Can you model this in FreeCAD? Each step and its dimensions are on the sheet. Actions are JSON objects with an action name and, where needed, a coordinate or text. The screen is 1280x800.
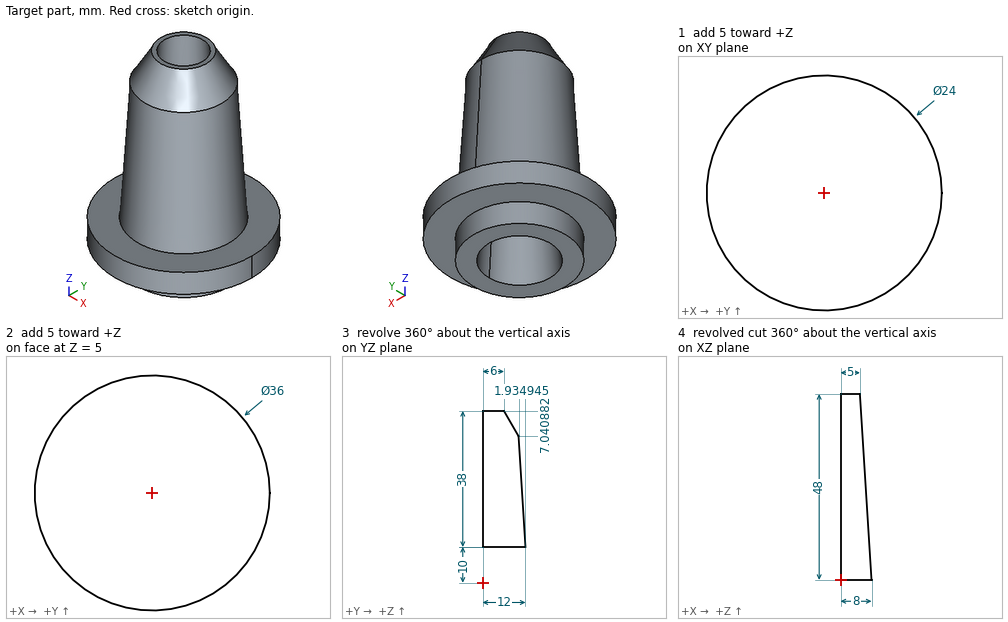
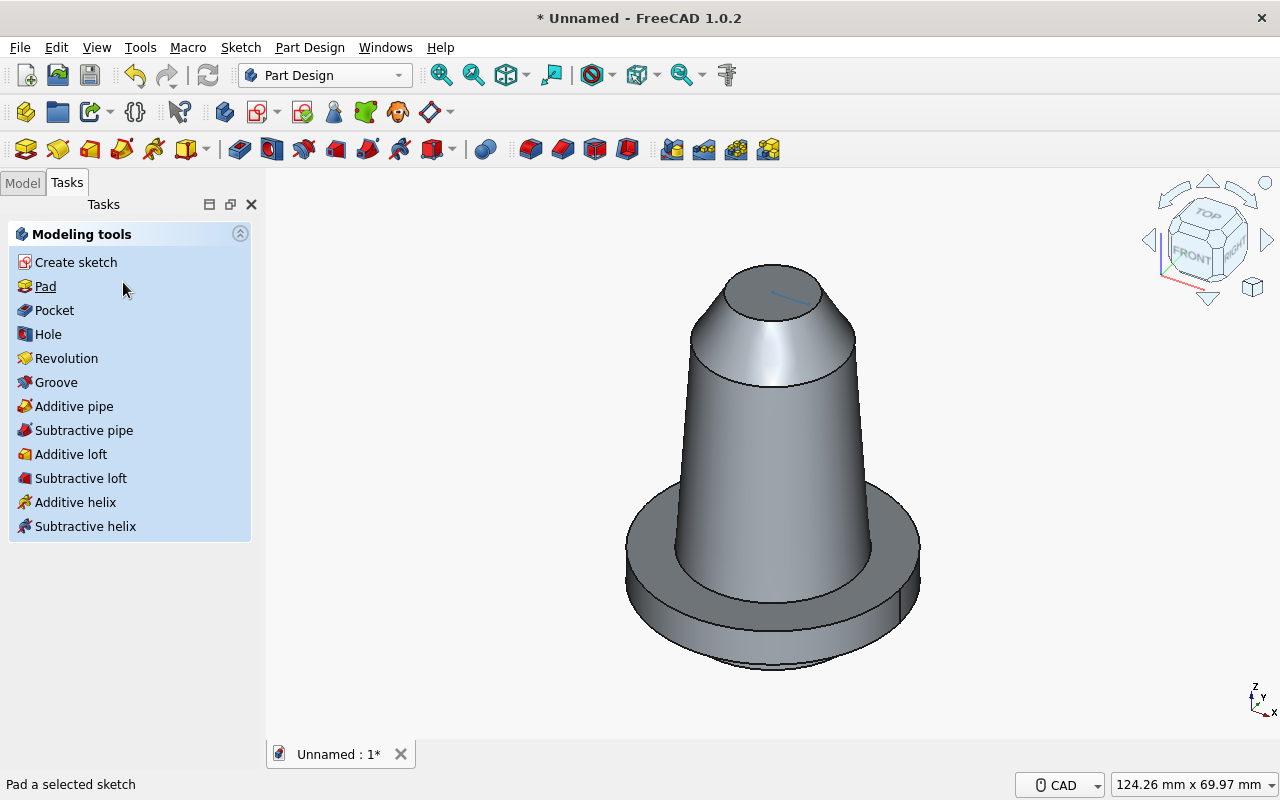
{"action": "left_click", "coordinate": [304, 150]}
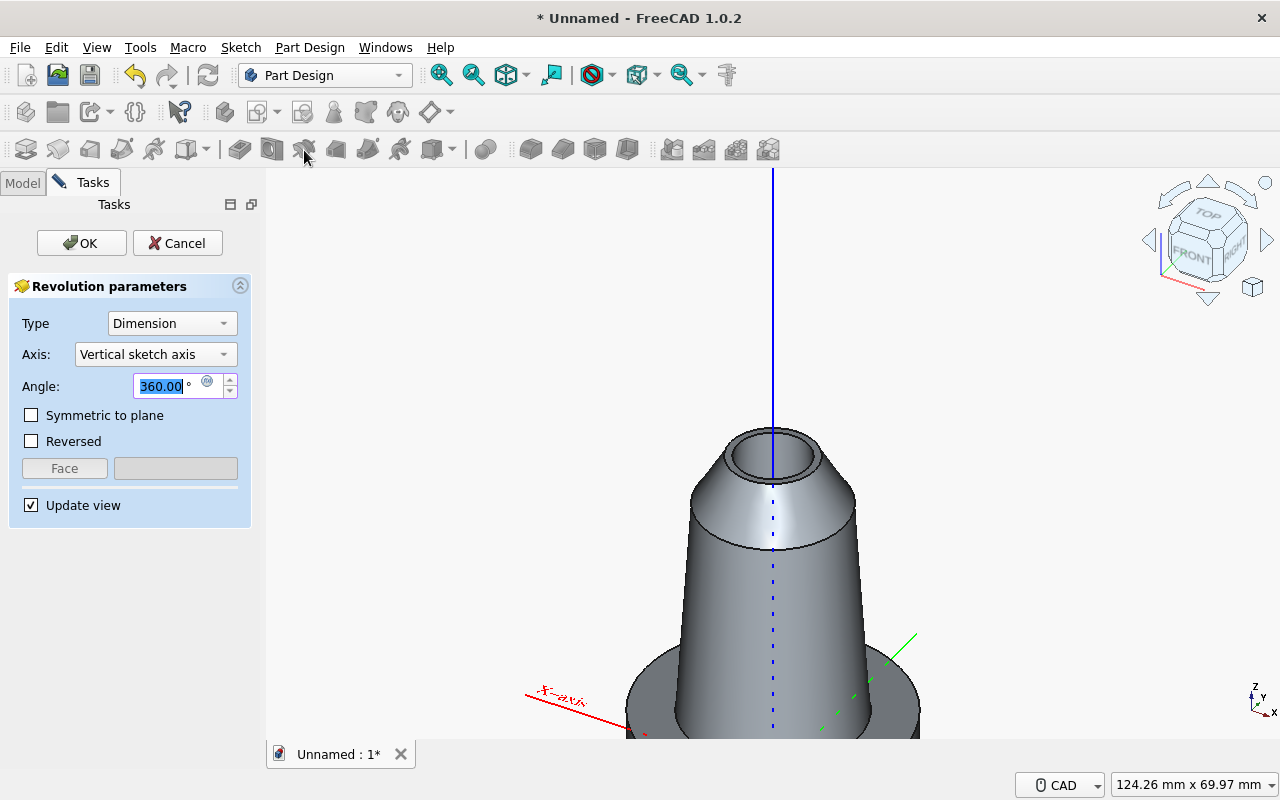
{"action": "left_click", "coordinate": [82, 243]}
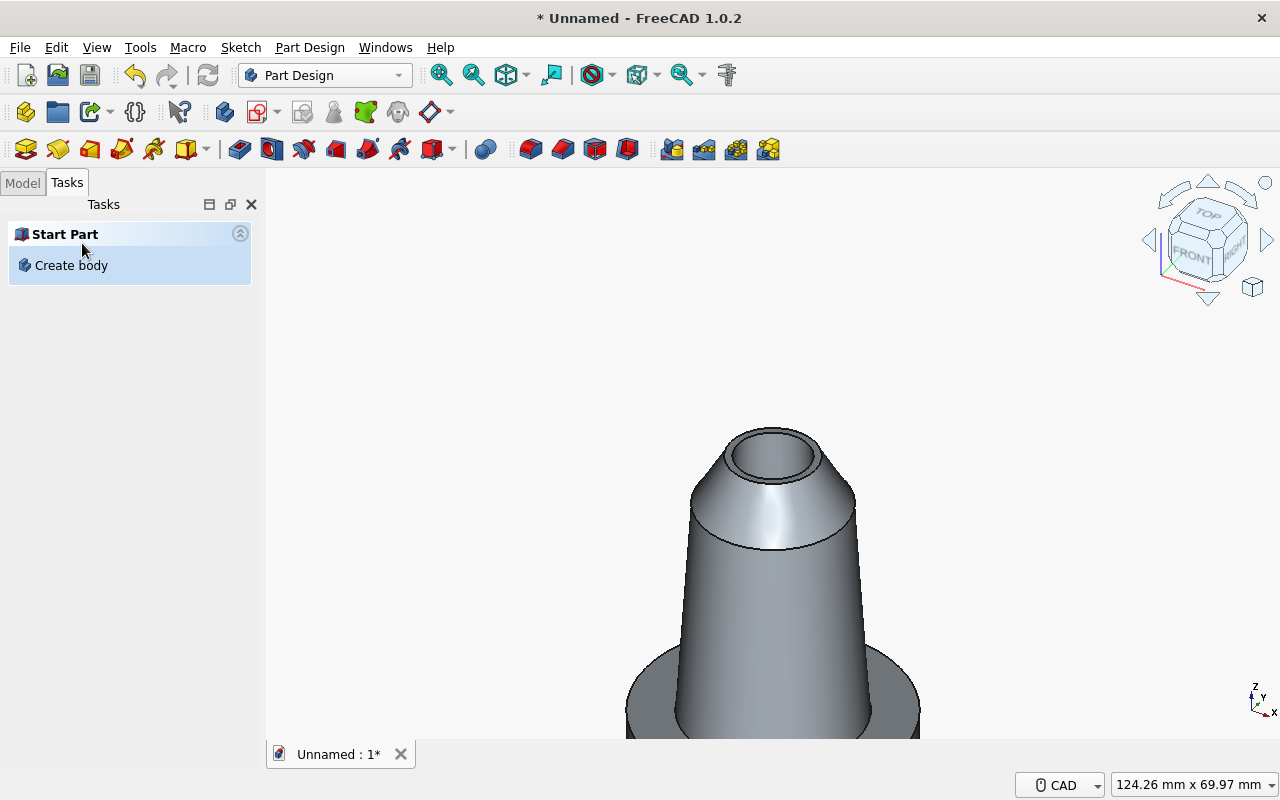
{"action": "key", "text": "0"}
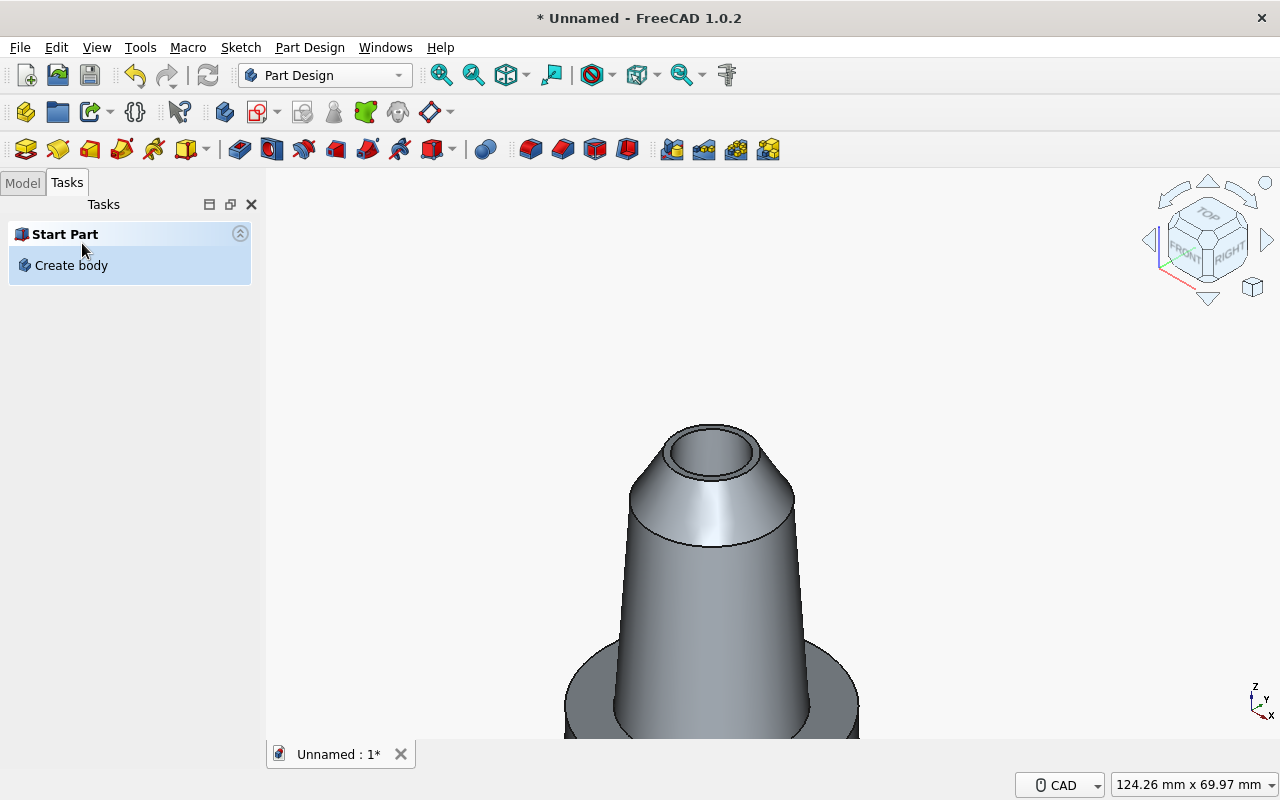
{"action": "left_click", "coordinate": [442, 76]}